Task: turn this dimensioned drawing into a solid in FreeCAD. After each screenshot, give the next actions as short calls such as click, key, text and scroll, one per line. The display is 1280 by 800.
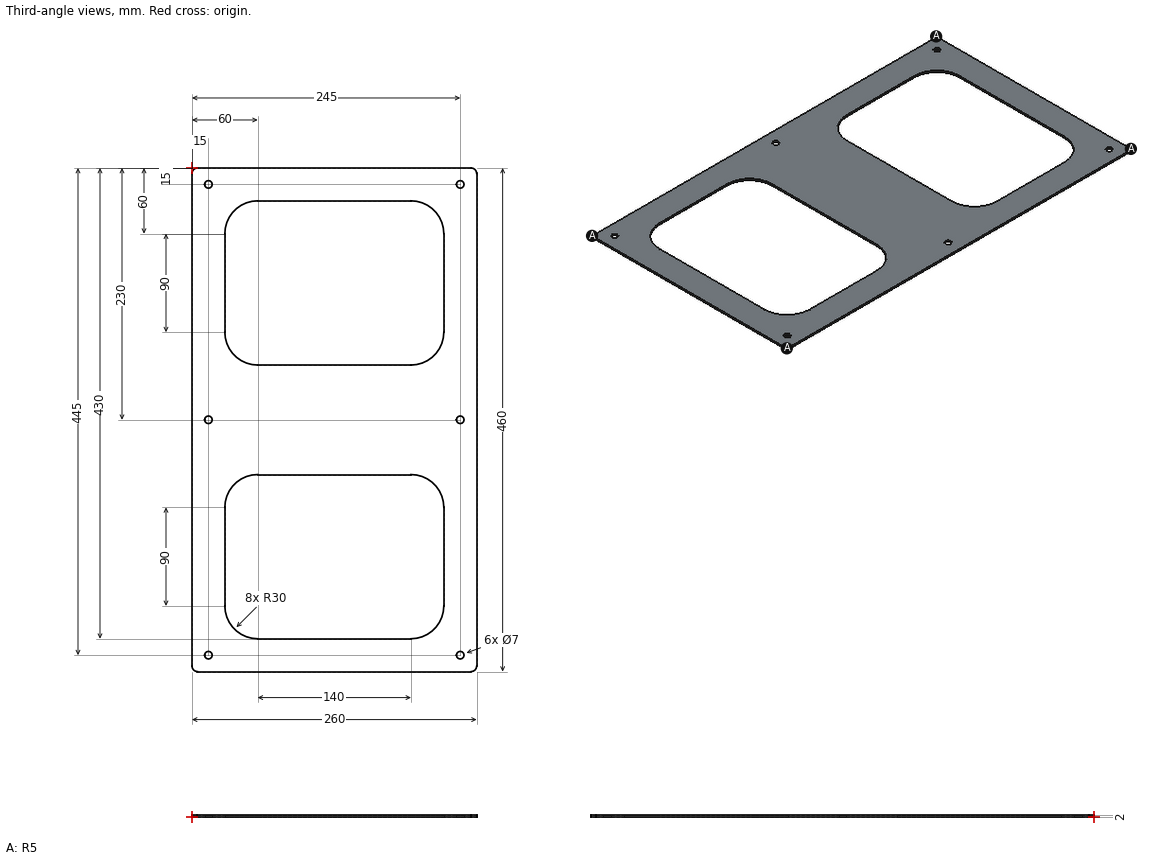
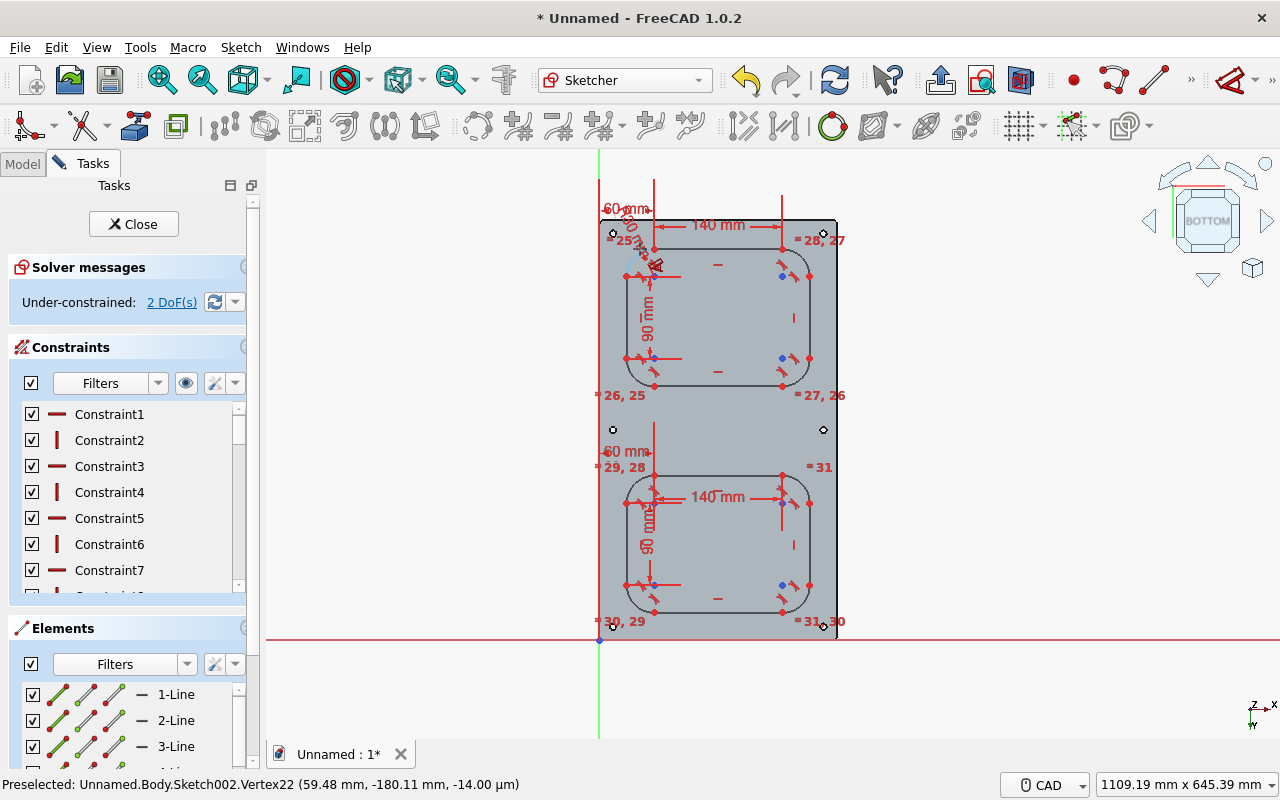
click(627, 585)
click(565, 613)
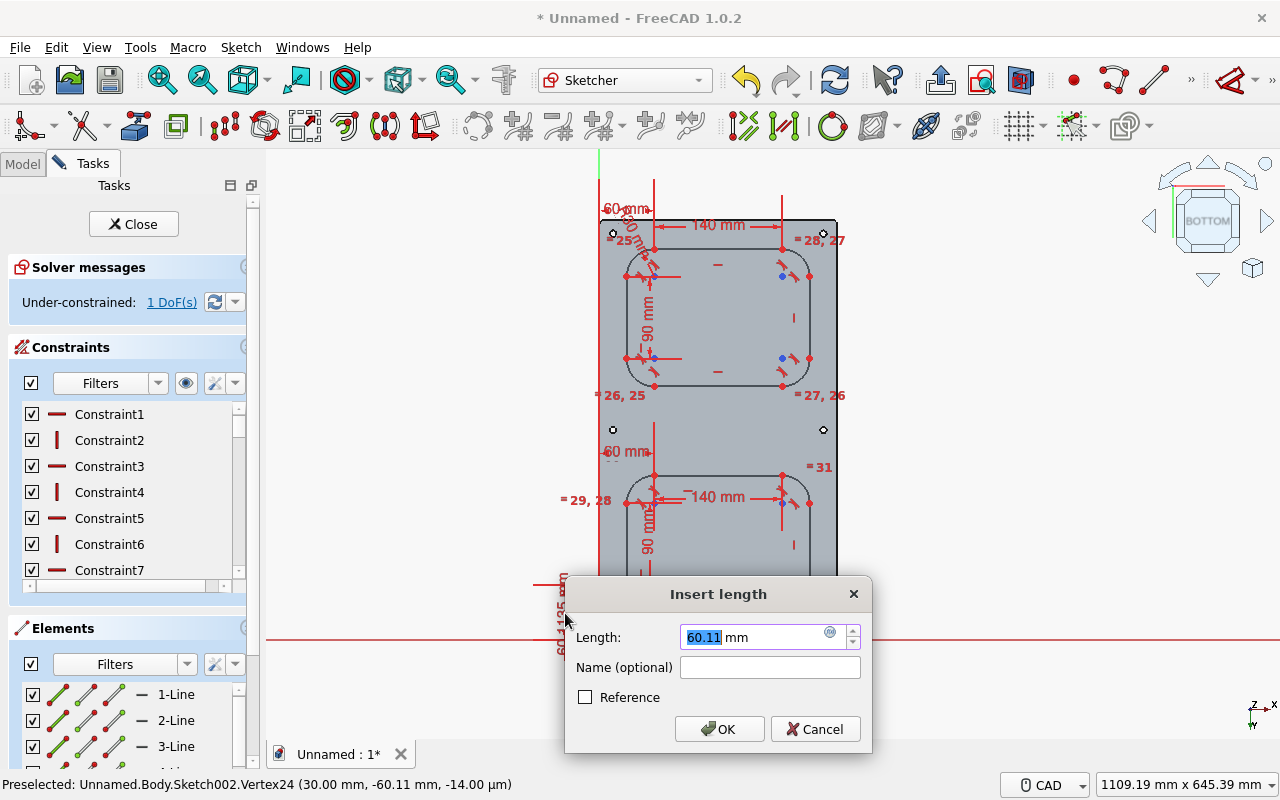
text(60)
key(Return)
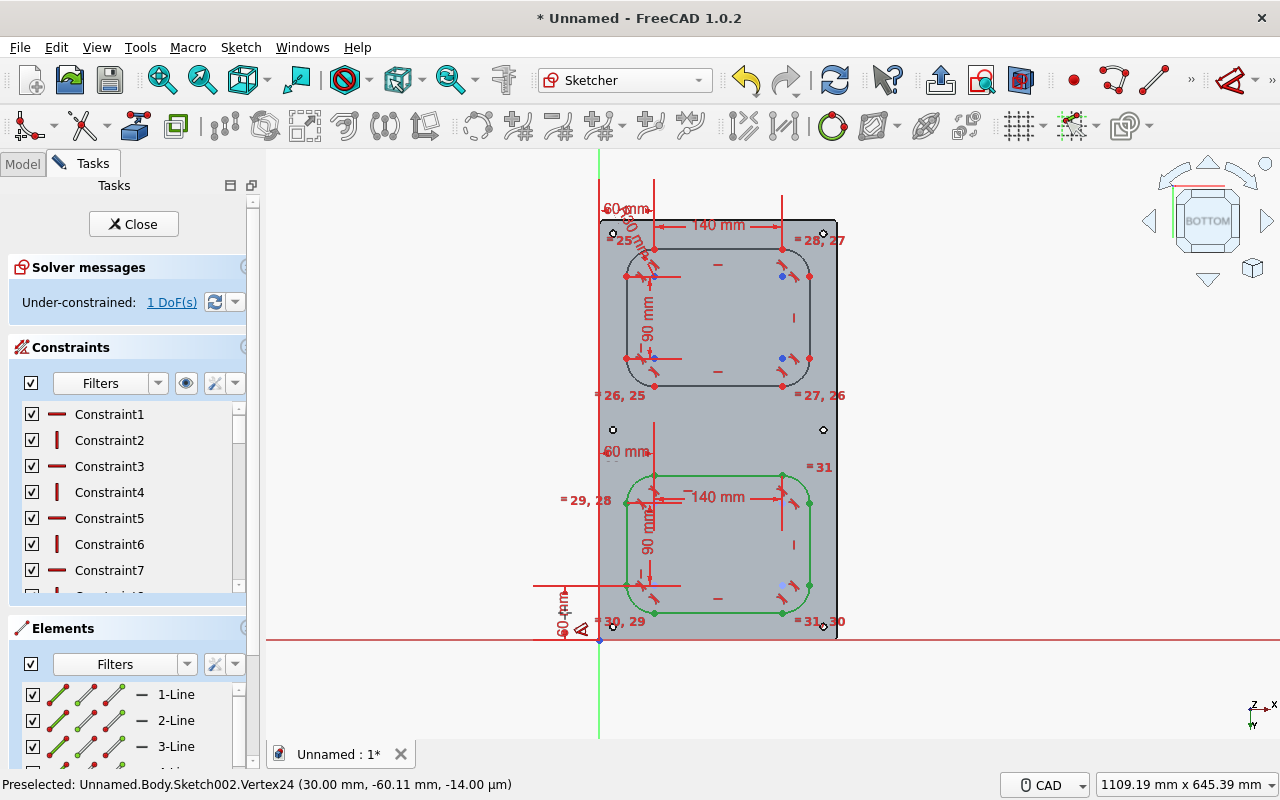
click(782, 249)
click(565, 355)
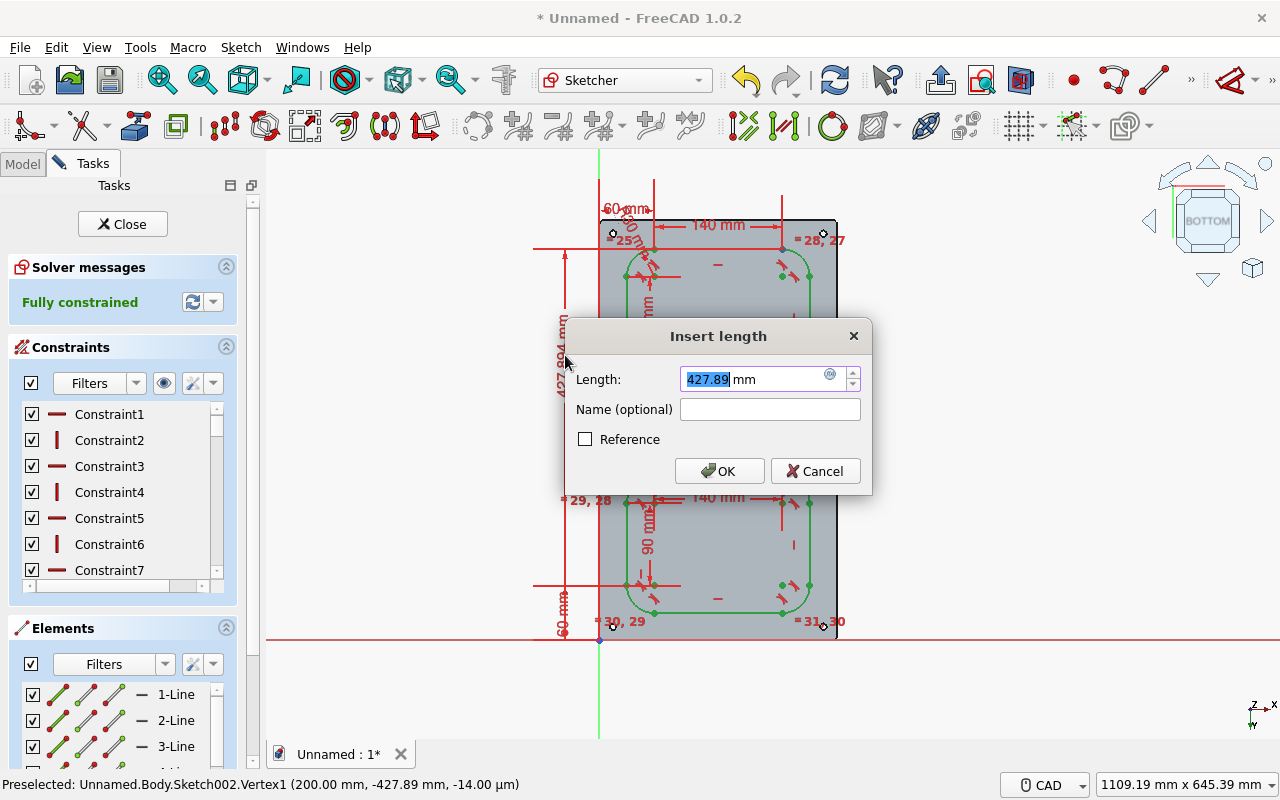
text(430)
key(Return)
key(Escape)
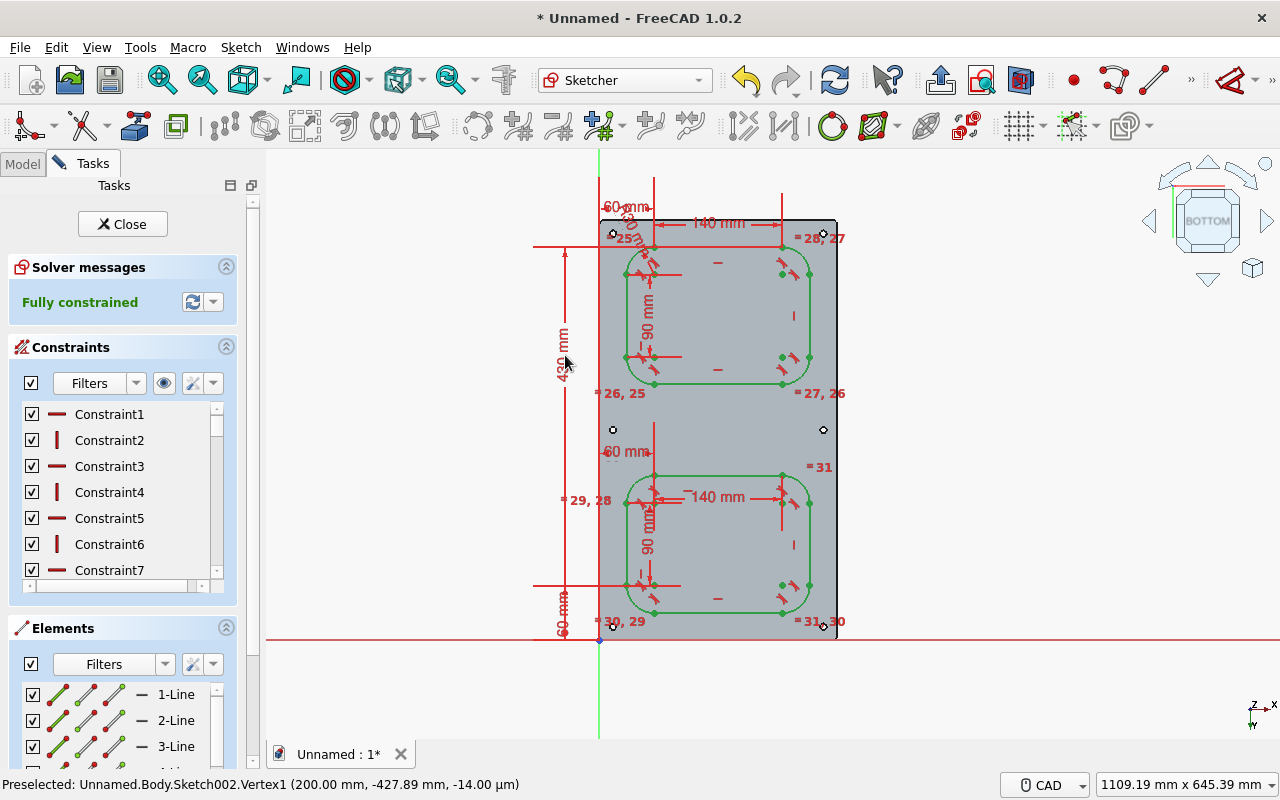
click(123, 224)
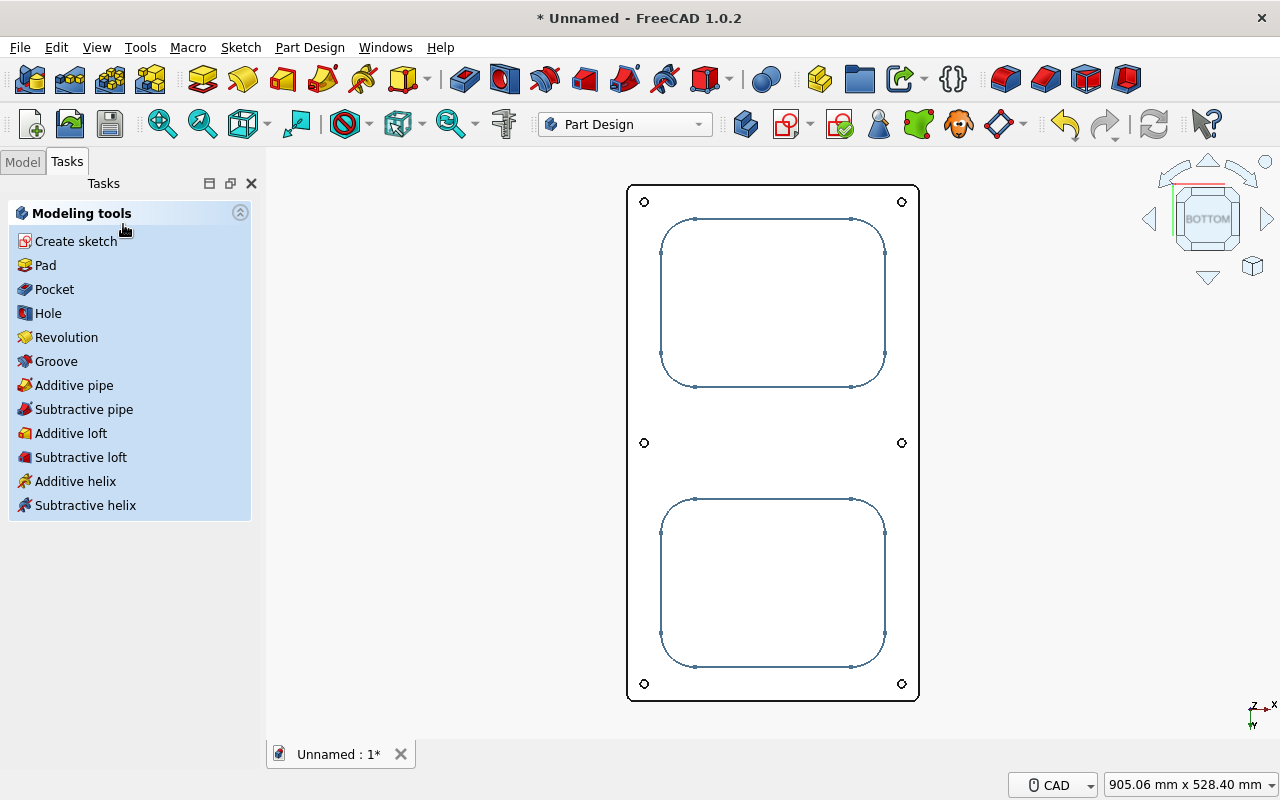
click(466, 80)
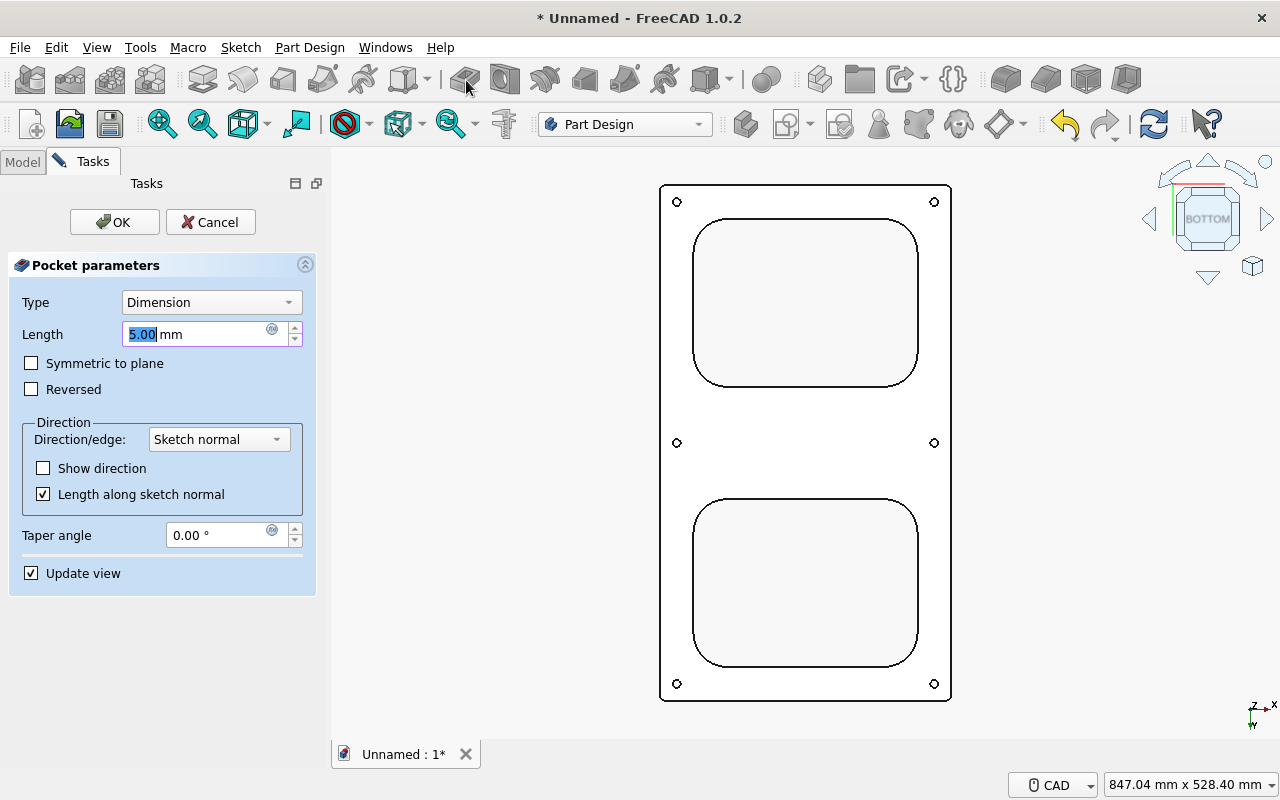
click(212, 302)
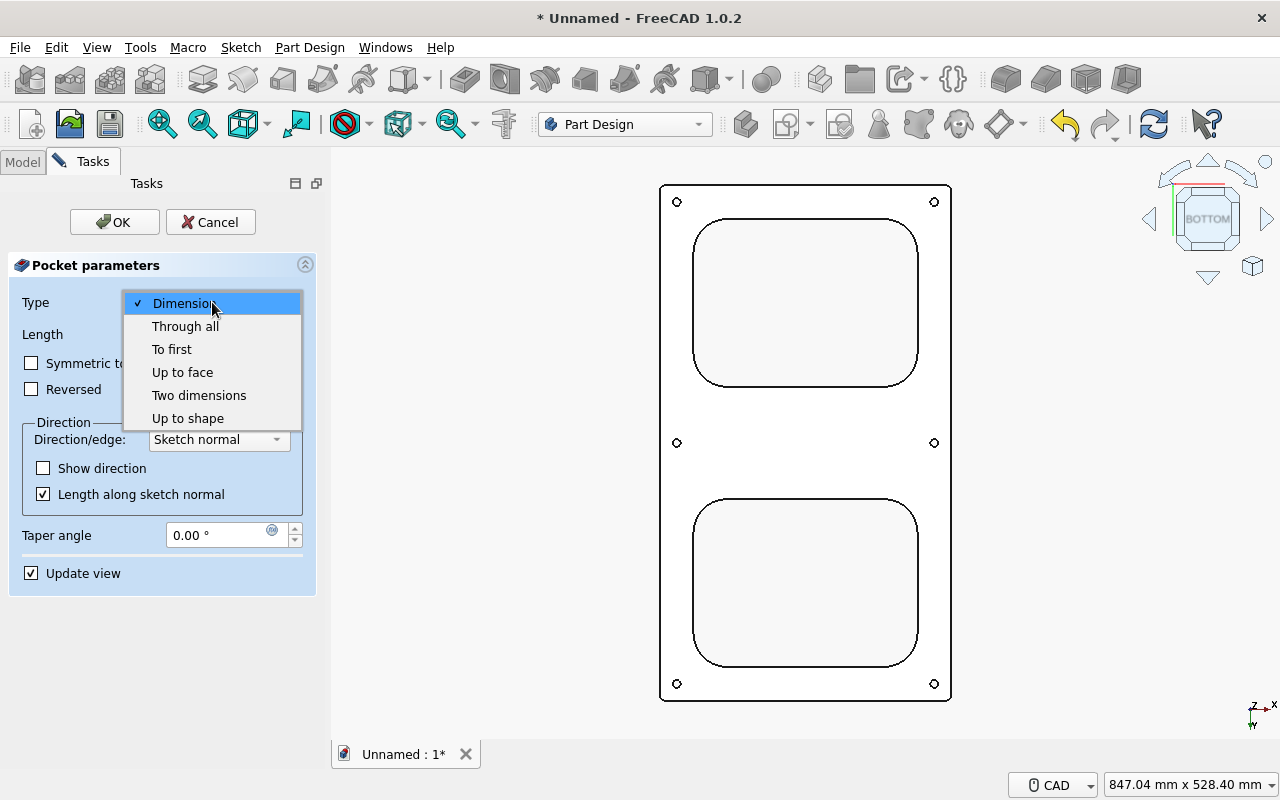
click(212, 326)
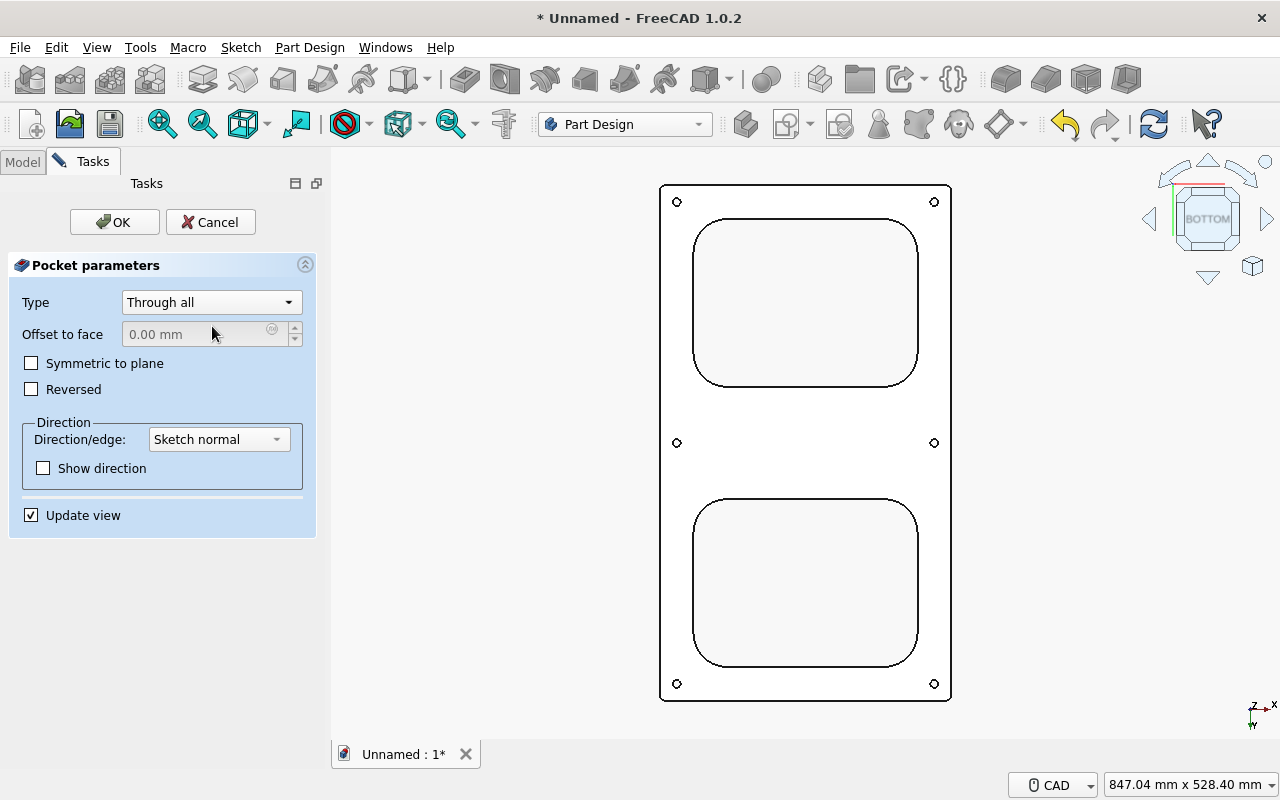
click(115, 222)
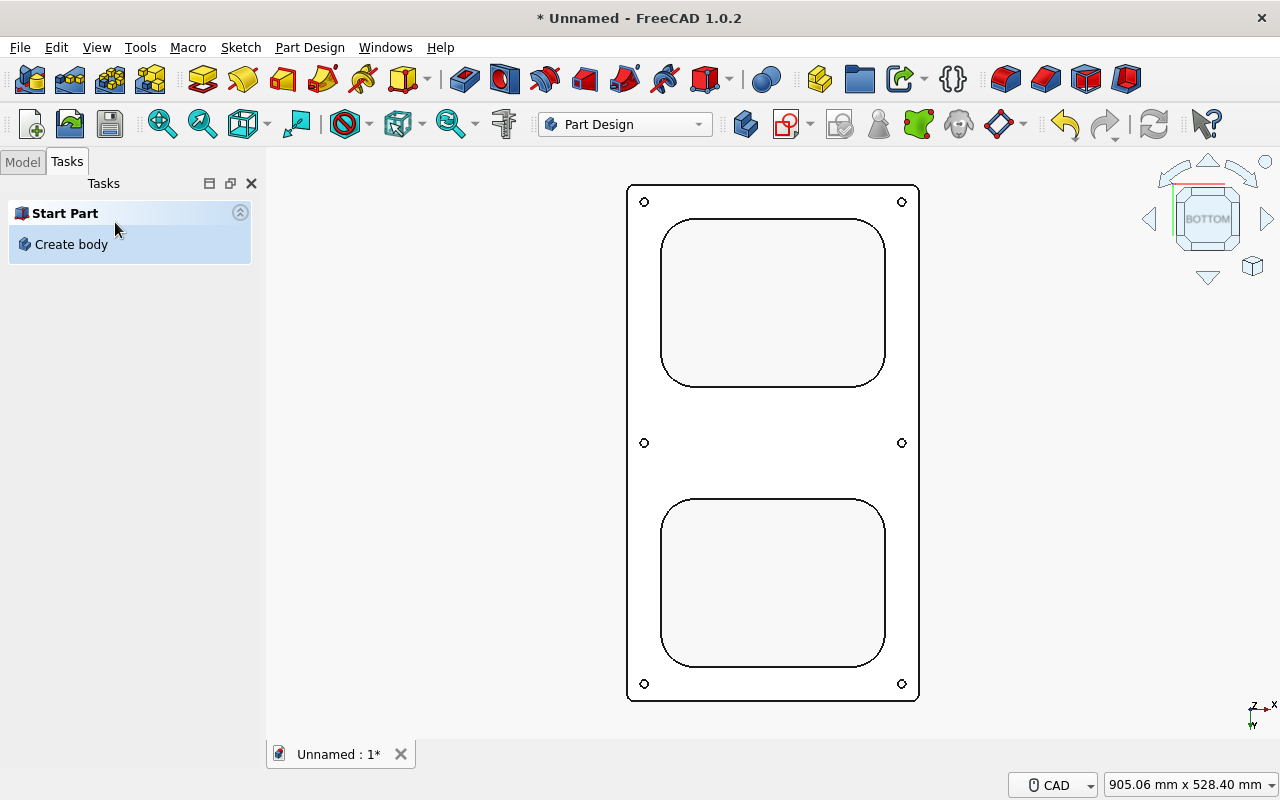
key(0)